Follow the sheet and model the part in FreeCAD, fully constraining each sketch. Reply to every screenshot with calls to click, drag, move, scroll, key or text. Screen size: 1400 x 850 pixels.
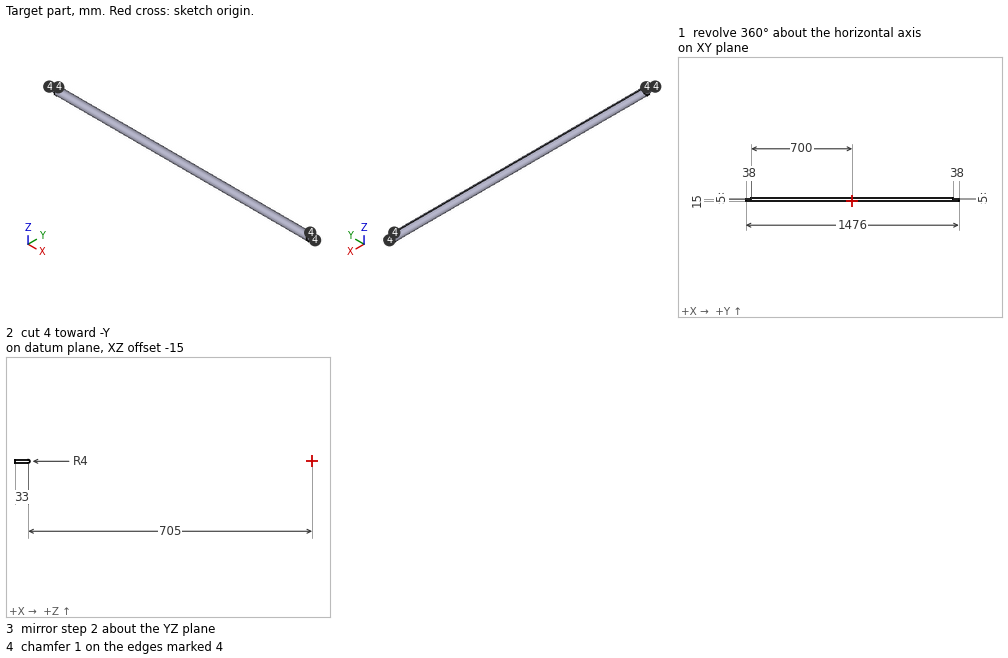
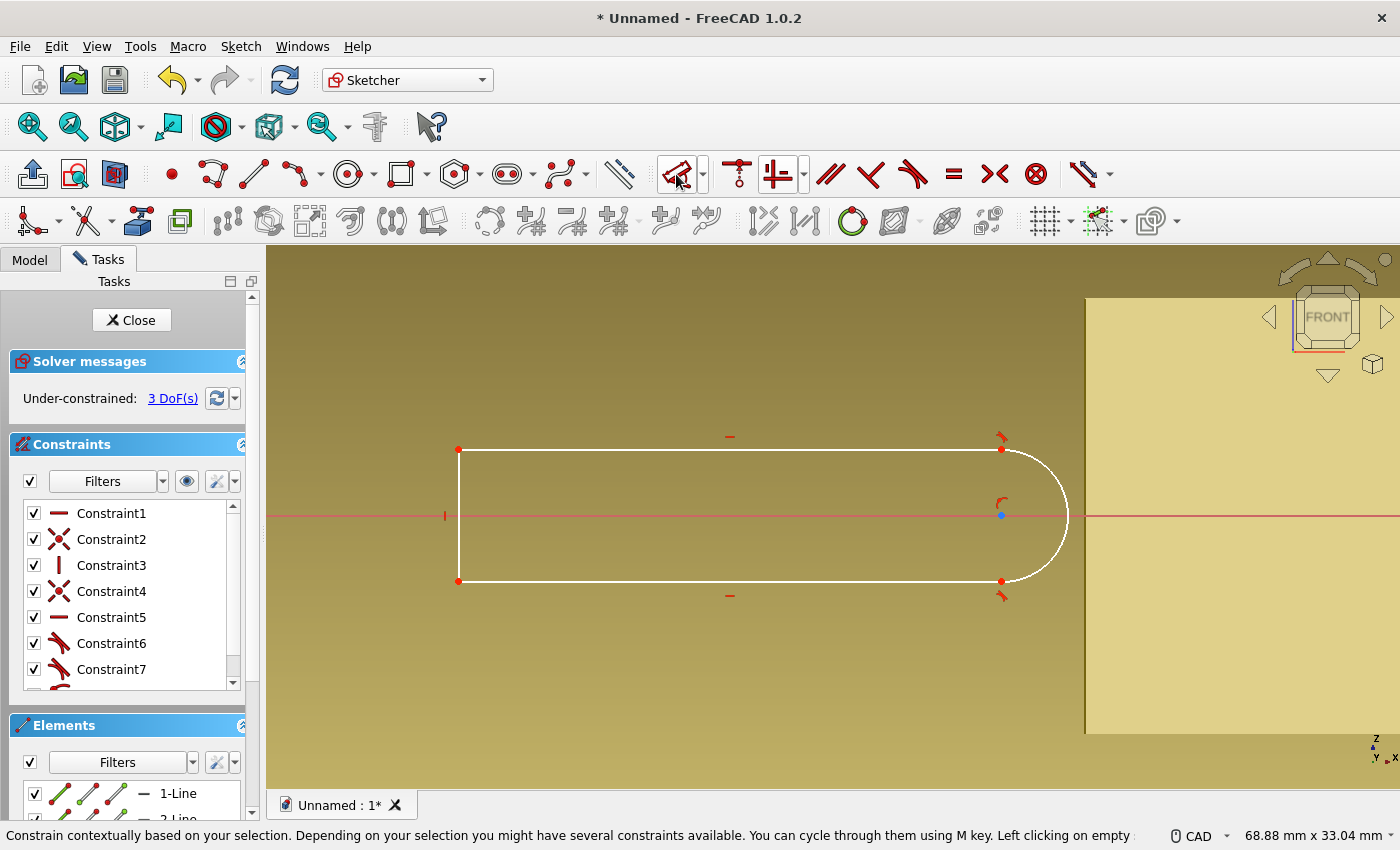
click(1055, 555)
click(1081, 574)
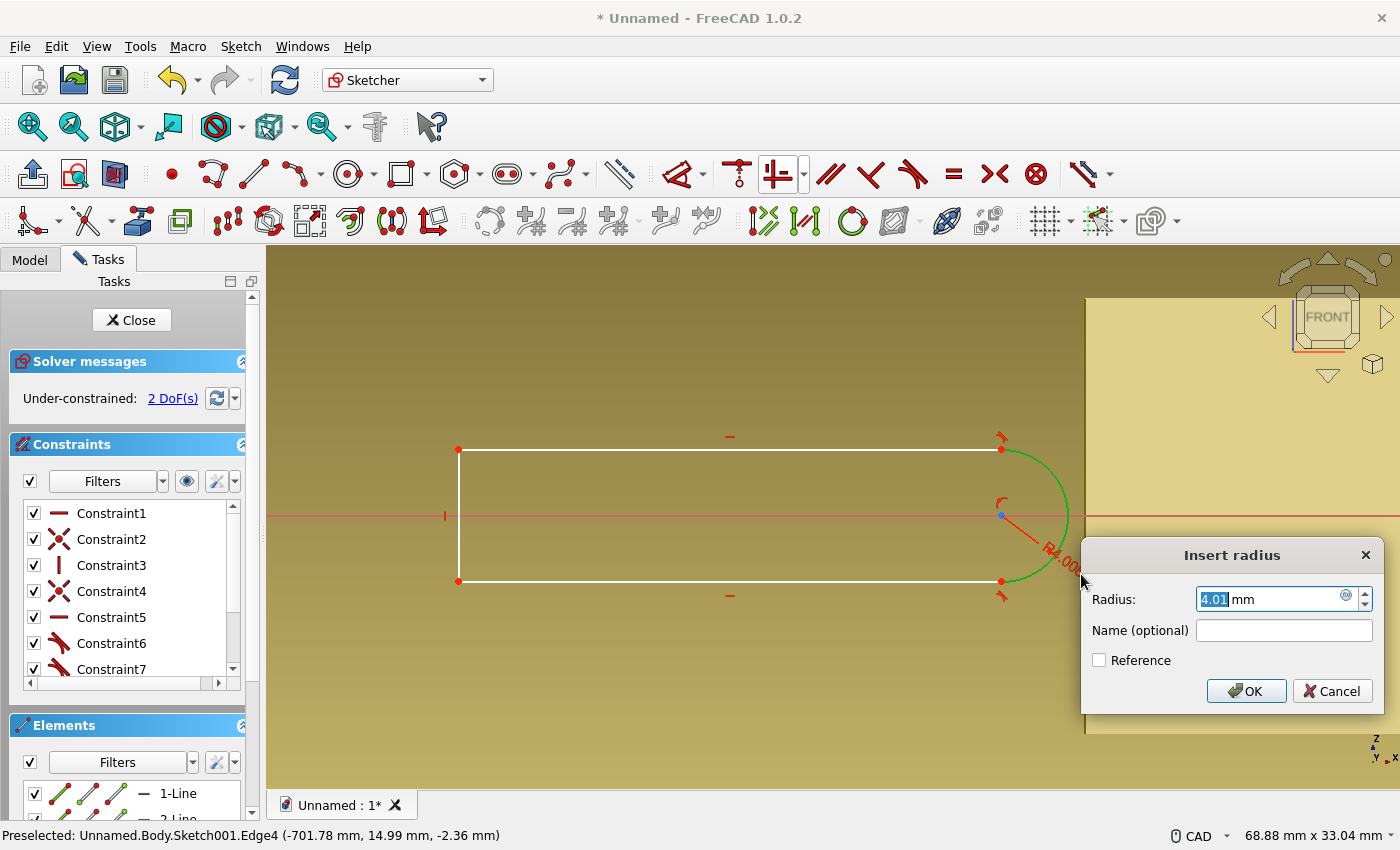
text(4)
key(Return)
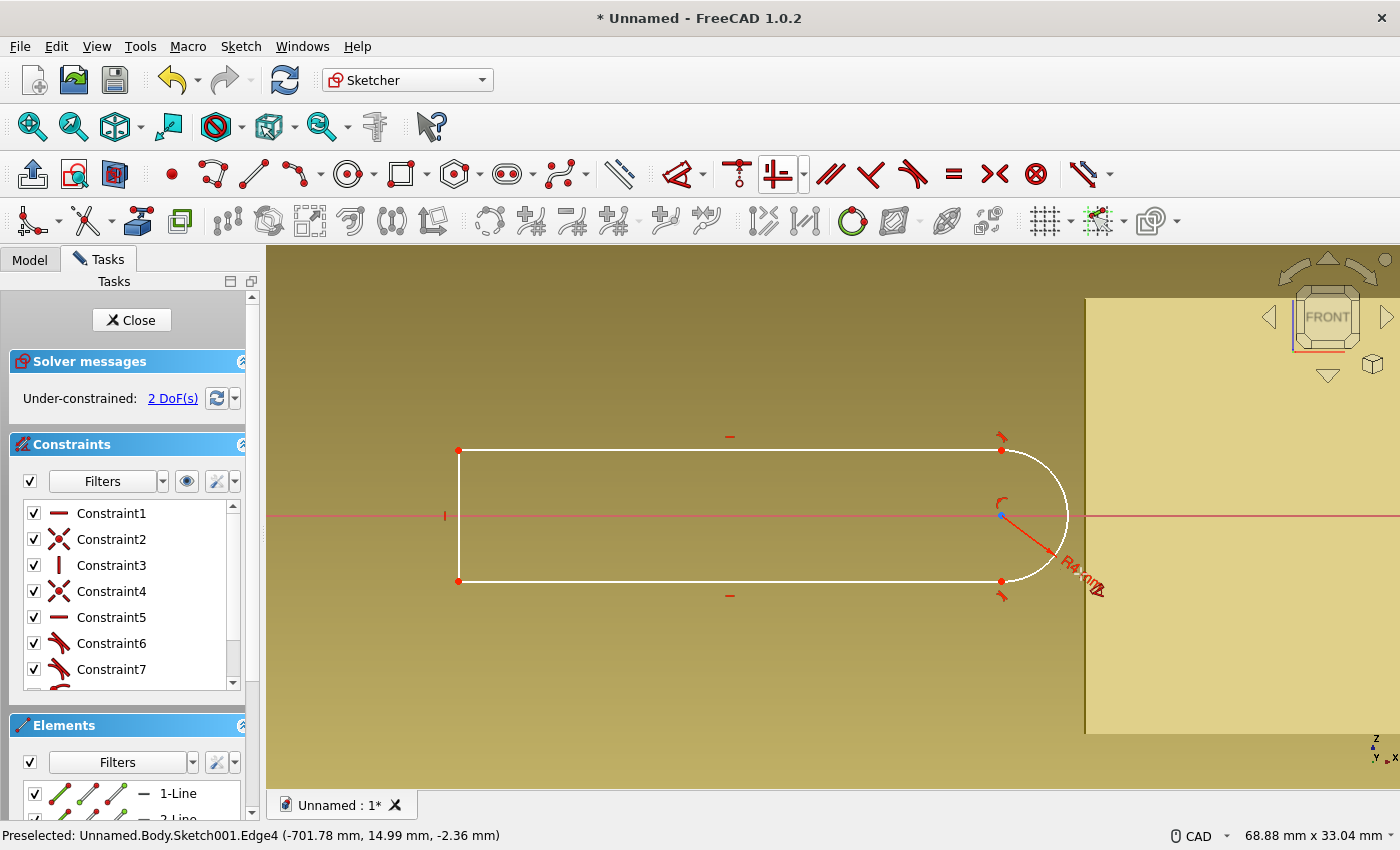
click(839, 582)
click(731, 616)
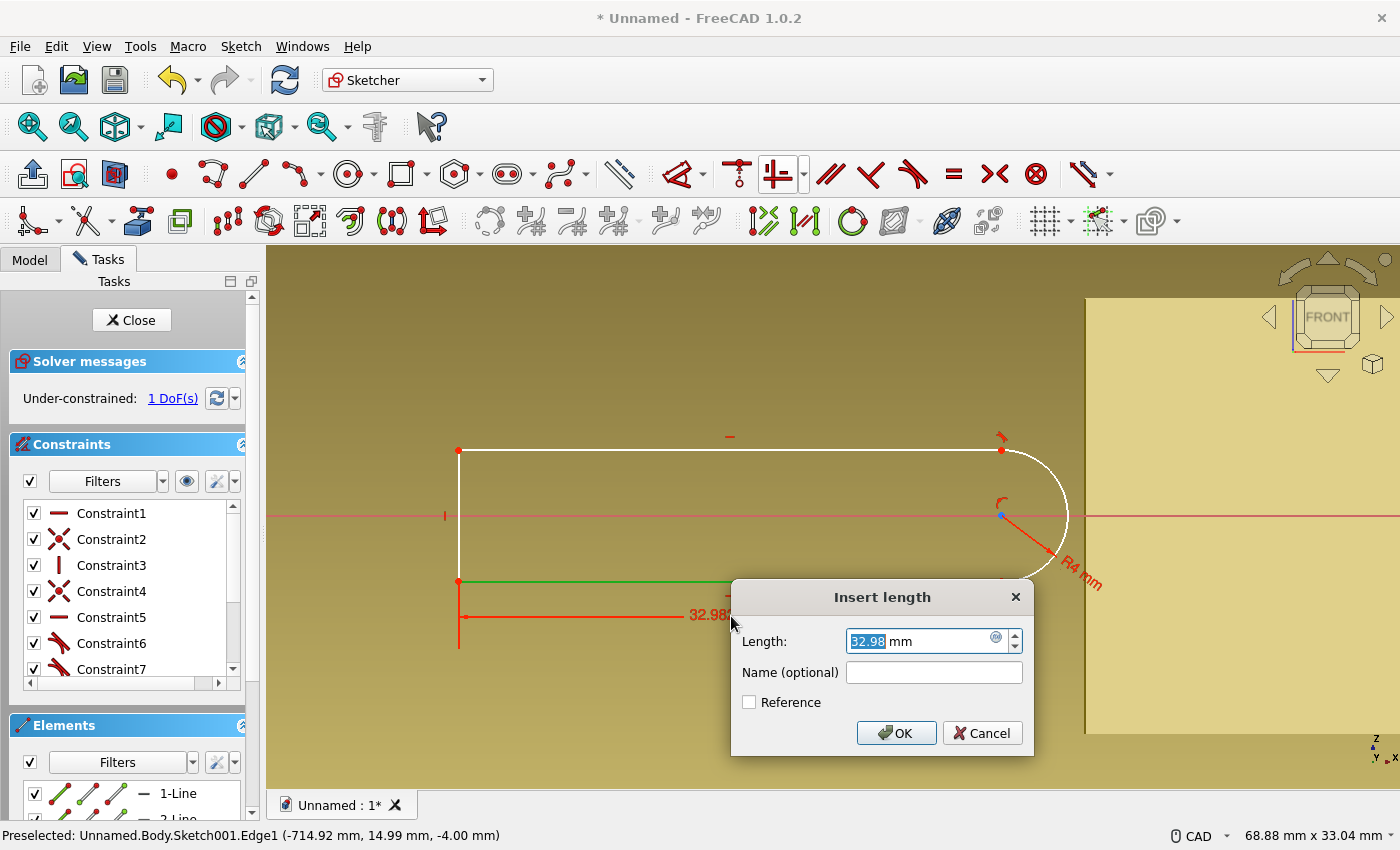
text(33)
key(Return)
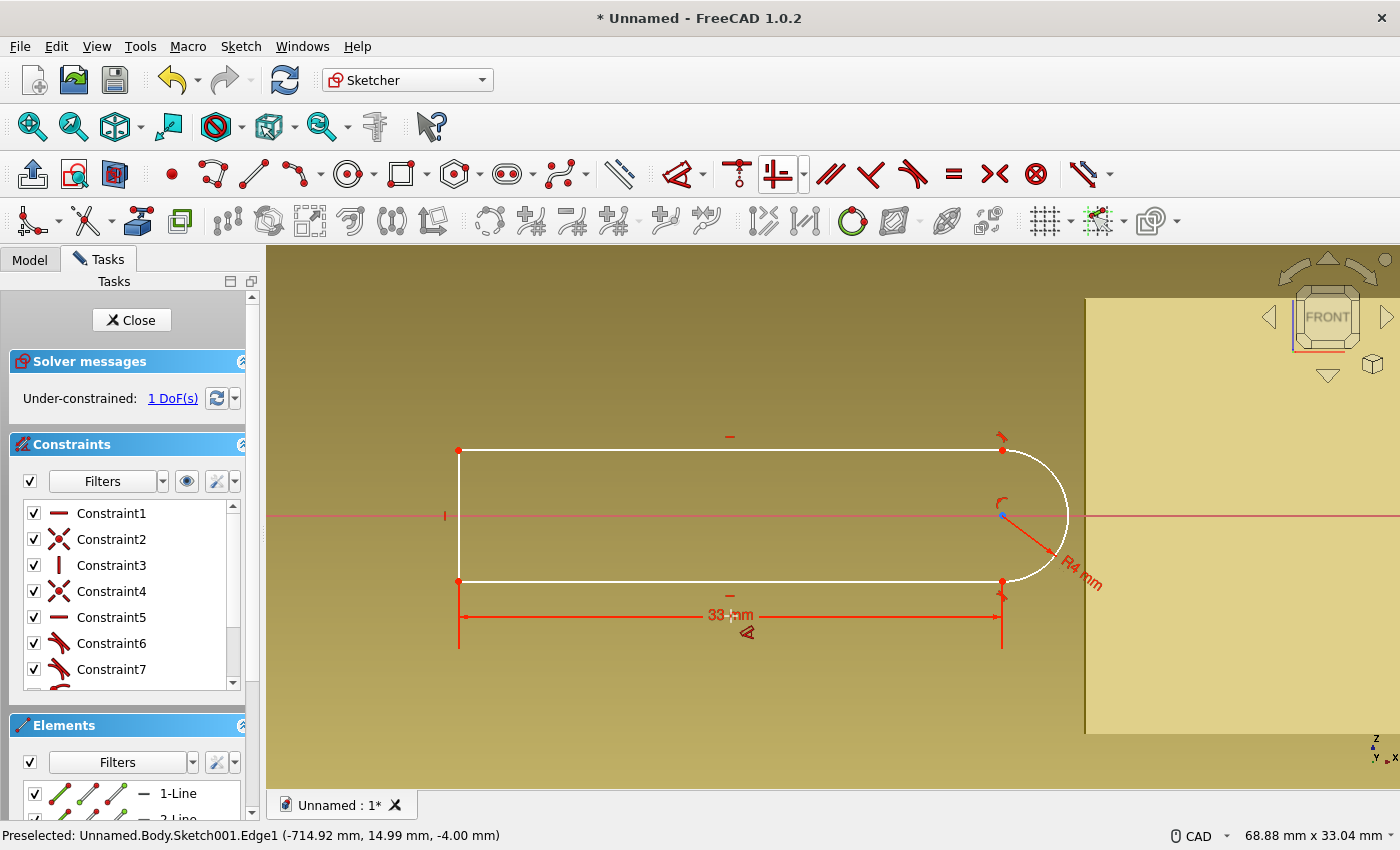
click(1002, 582)
click(1119, 616)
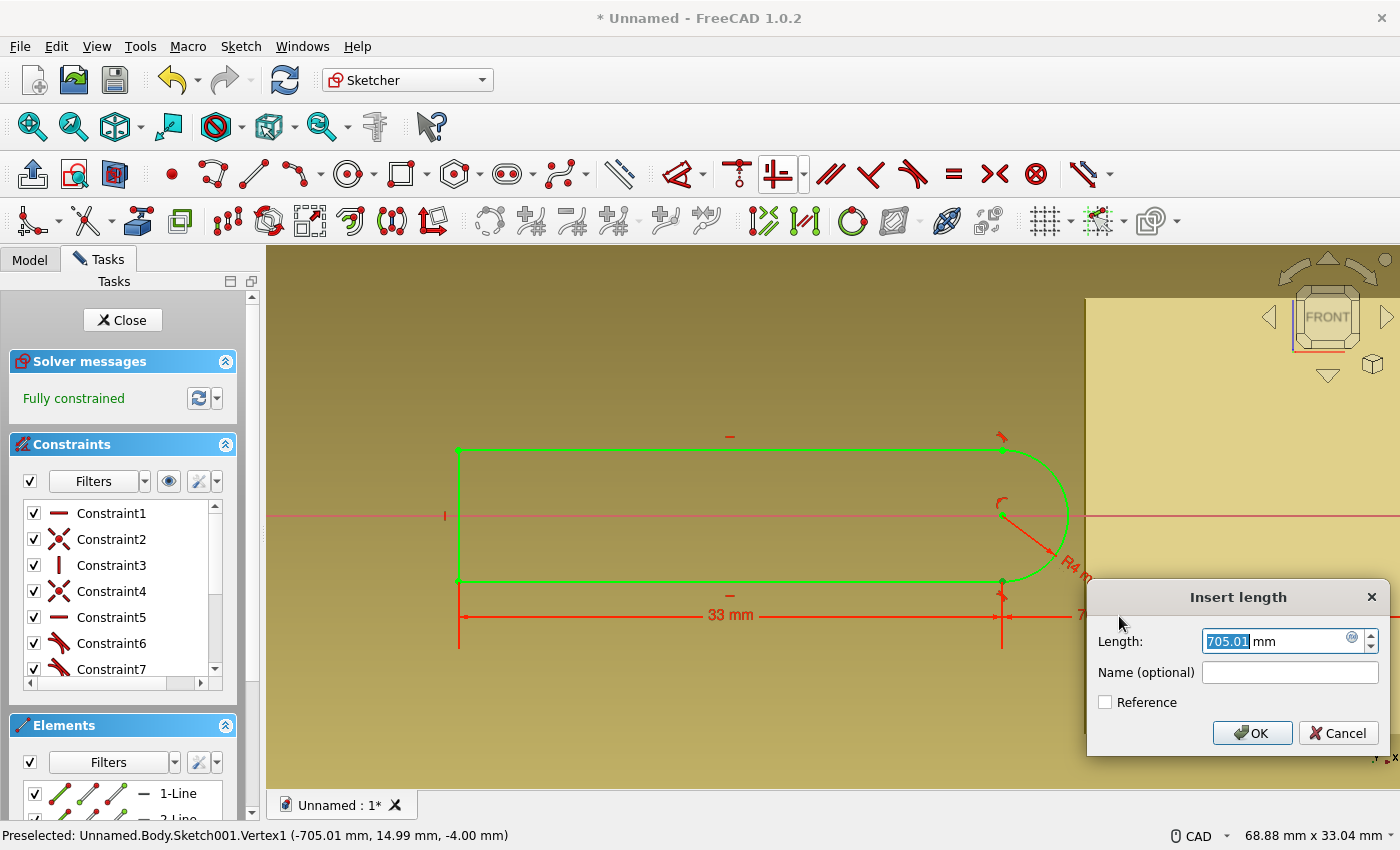
text(705)
key(Return)
key(Escape)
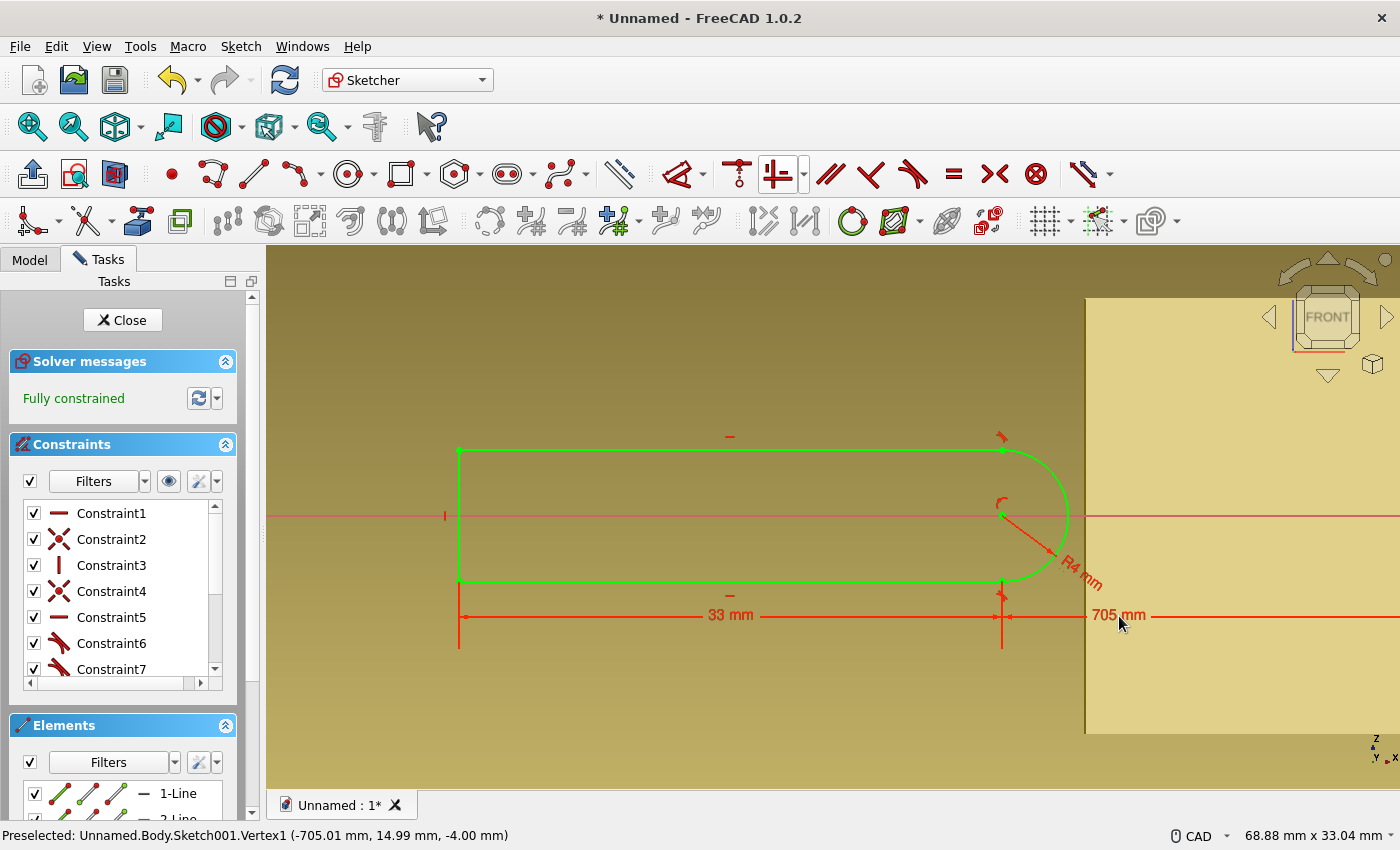
click(123, 320)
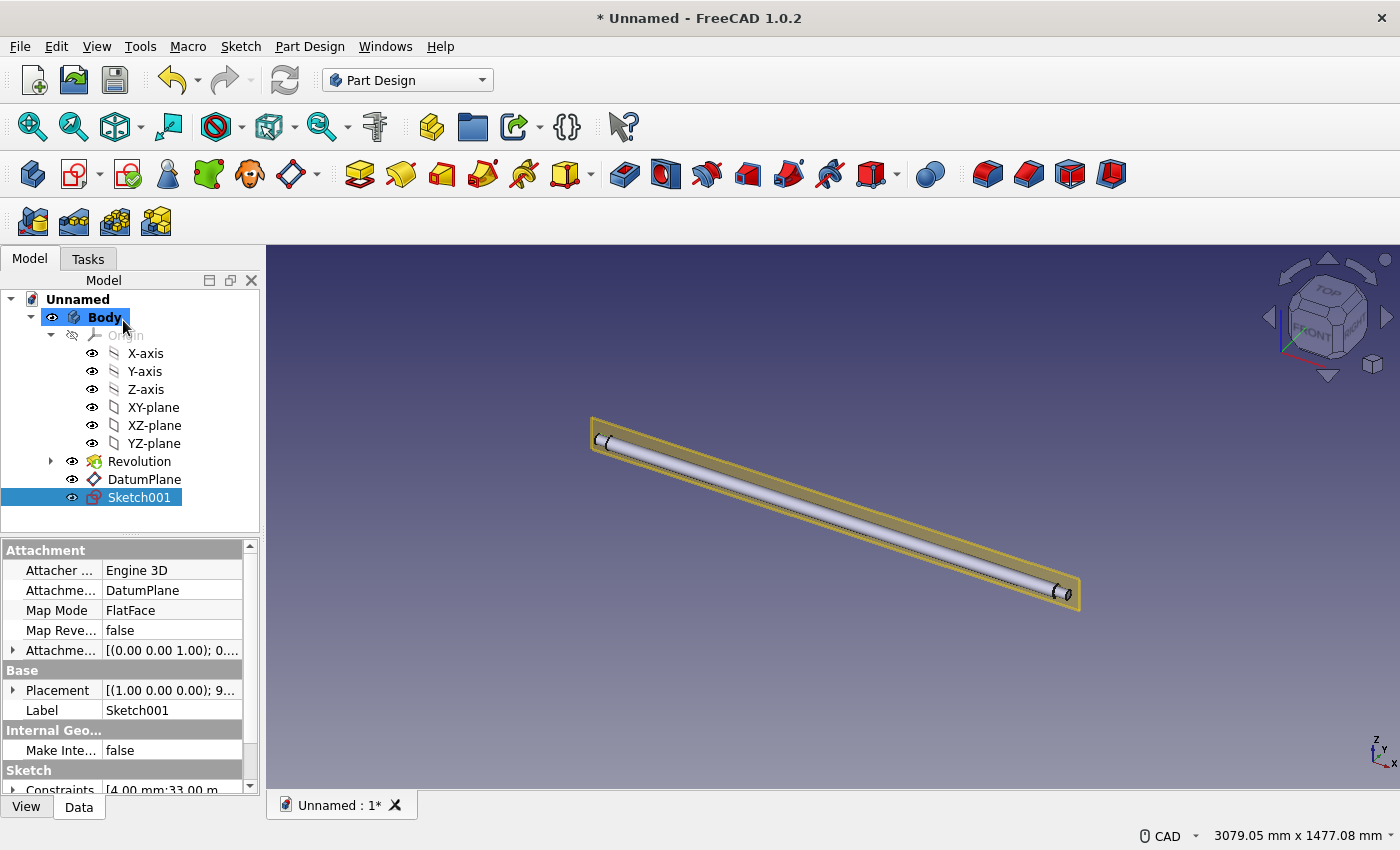
click(625, 174)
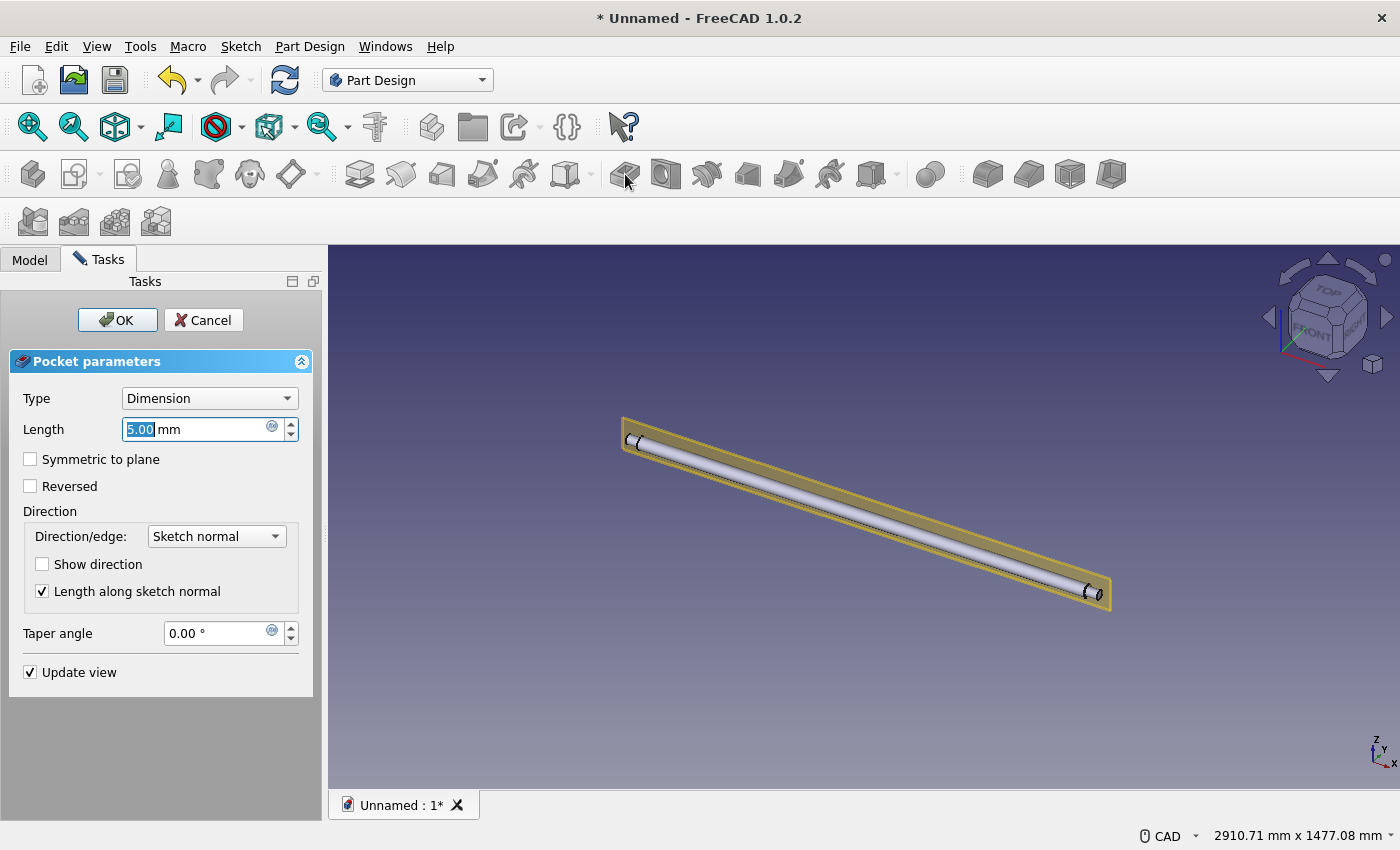
text(4)
key(Tab)